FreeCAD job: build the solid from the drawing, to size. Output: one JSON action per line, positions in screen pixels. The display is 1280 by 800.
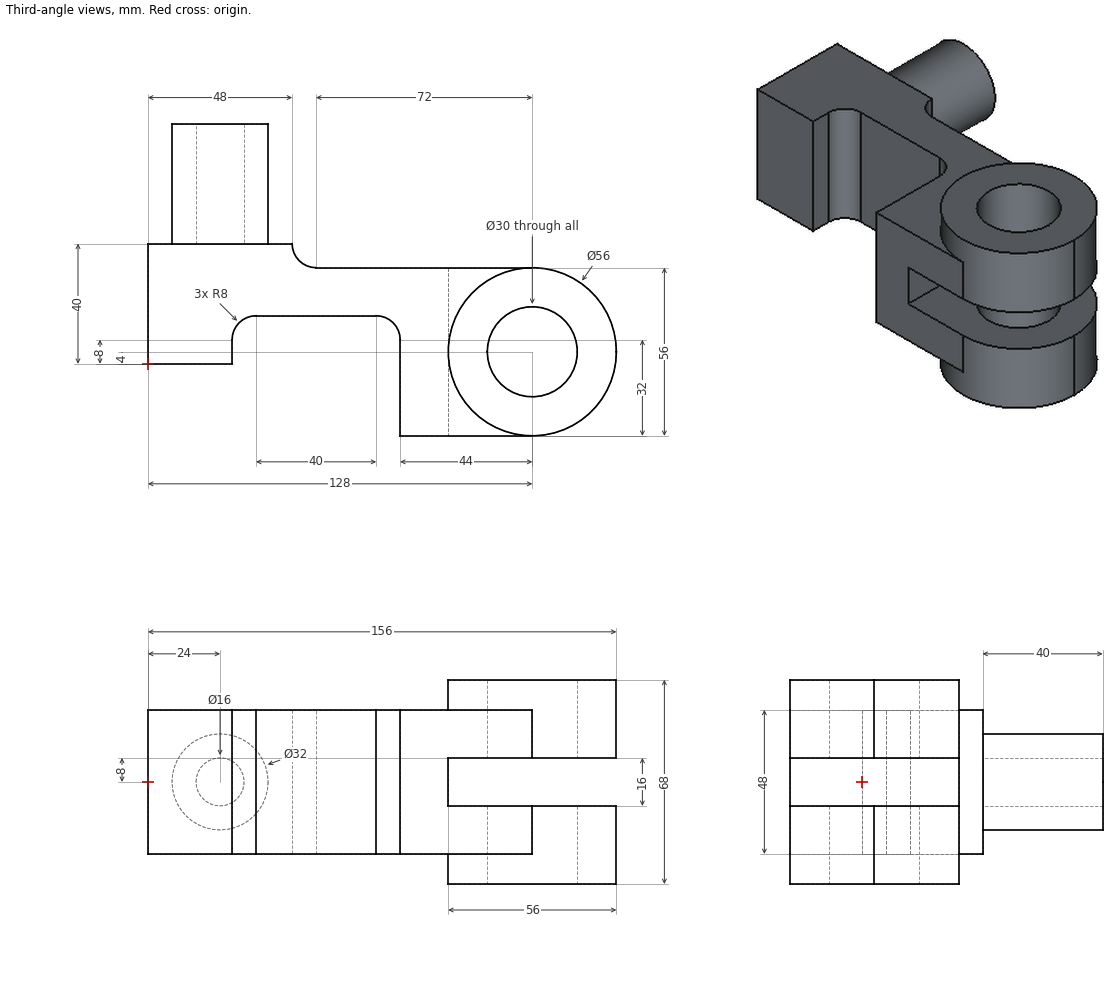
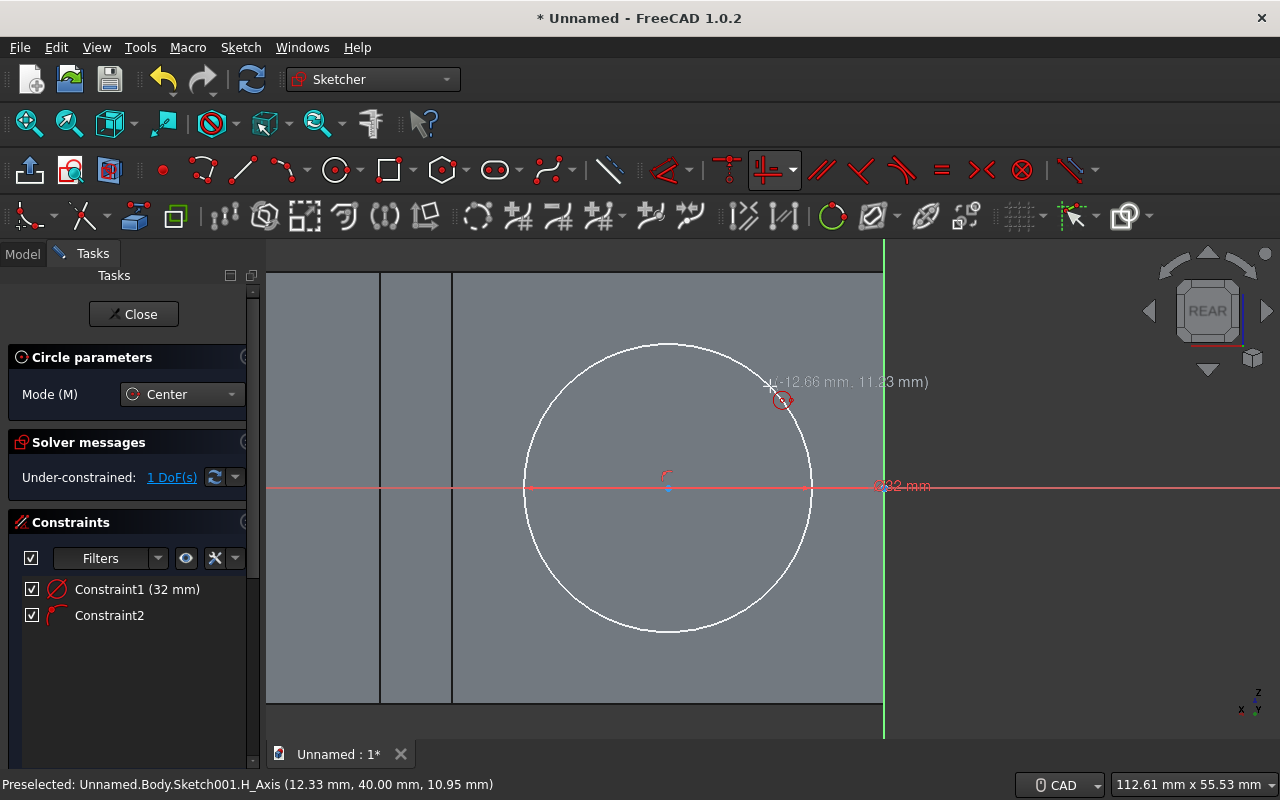
{"action": "left_click", "coordinate": [668, 488]}
{"action": "mouse_move", "coordinate": [719, 437]}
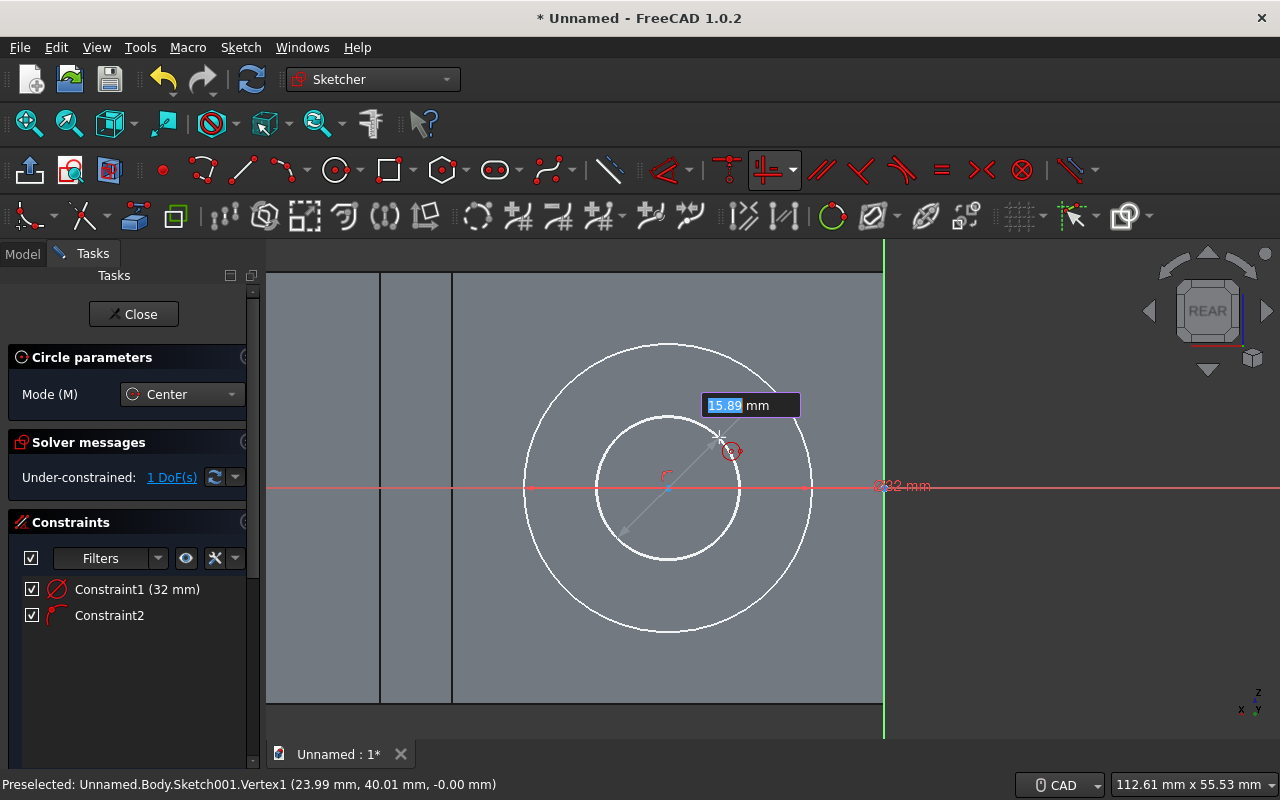
{"action": "type", "text": "16"}
{"action": "key", "text": "Return"}
{"action": "key", "text": "Escape"}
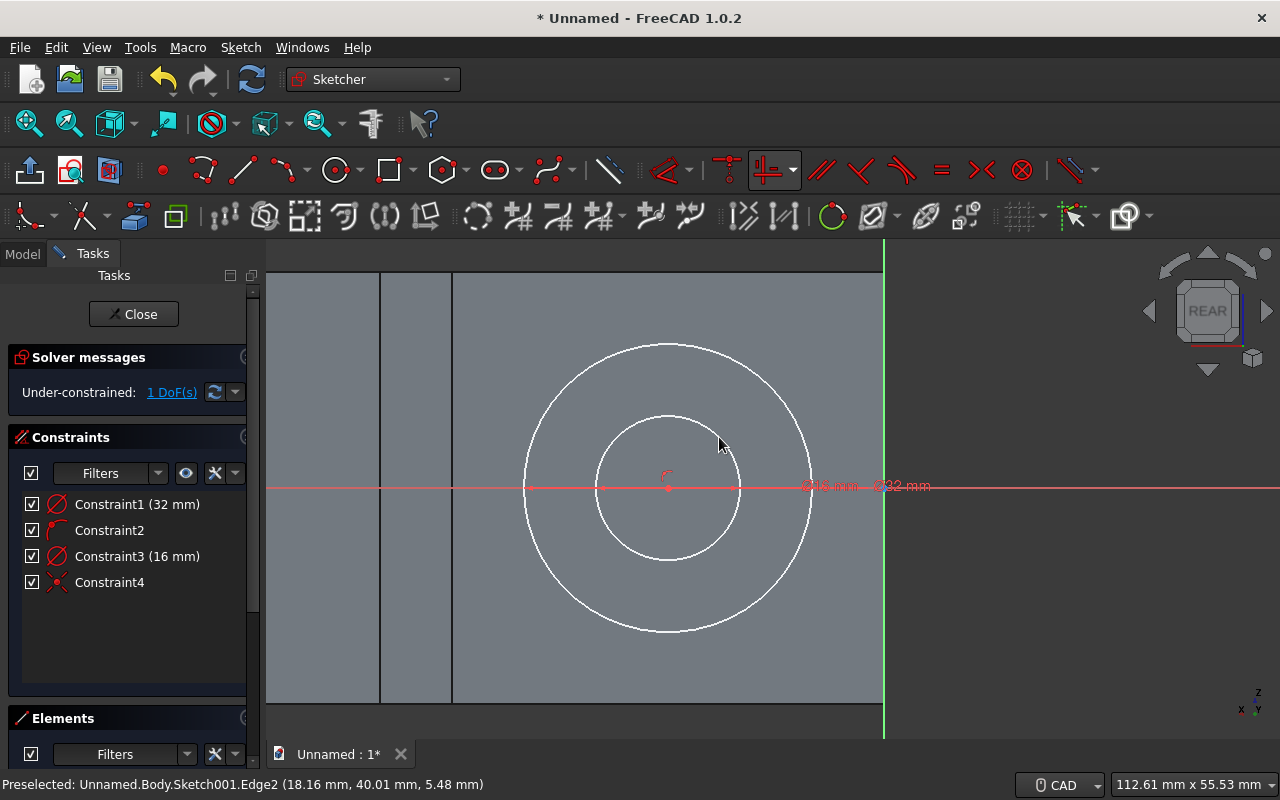
{"action": "left_click", "coordinate": [664, 170]}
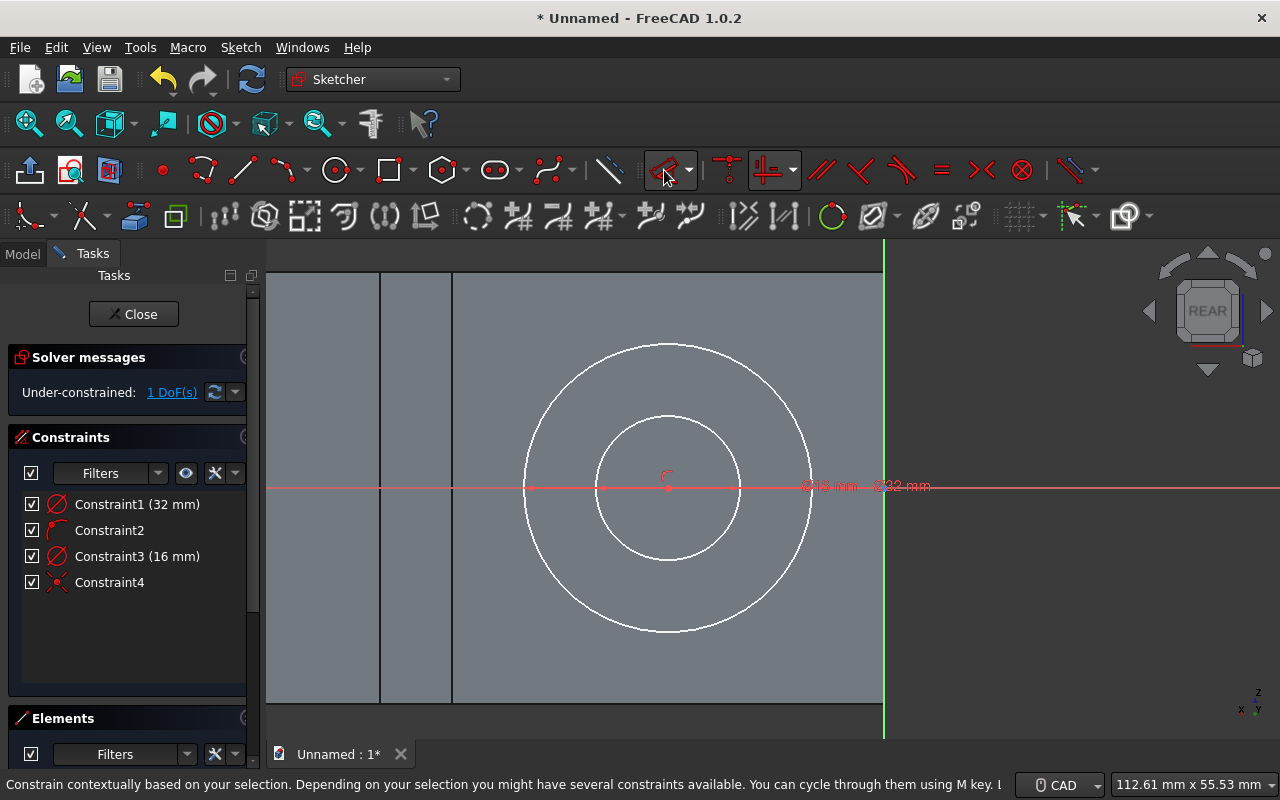
{"action": "left_click", "coordinate": [668, 488]}
{"action": "left_click", "coordinate": [776, 522]}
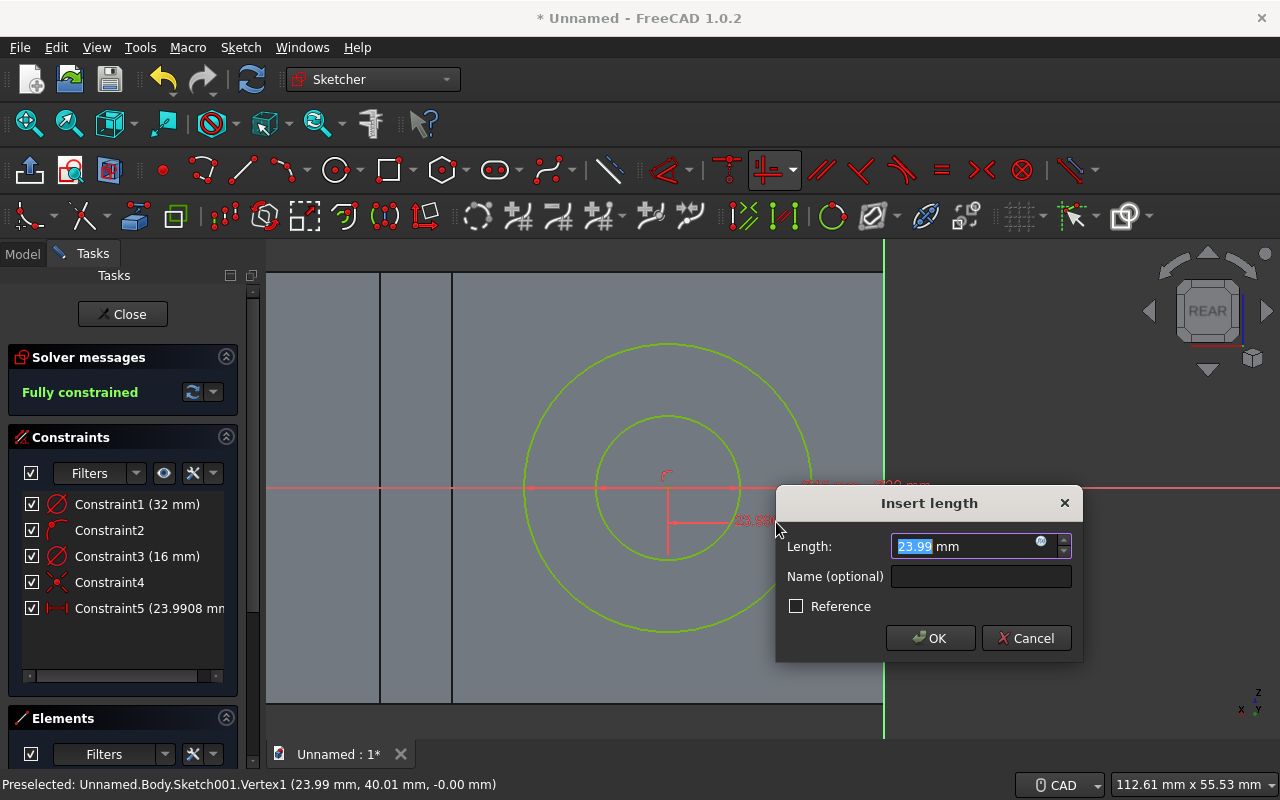
{"action": "type", "text": "24"}
{"action": "key", "text": "Return"}
{"action": "key", "text": "Escape"}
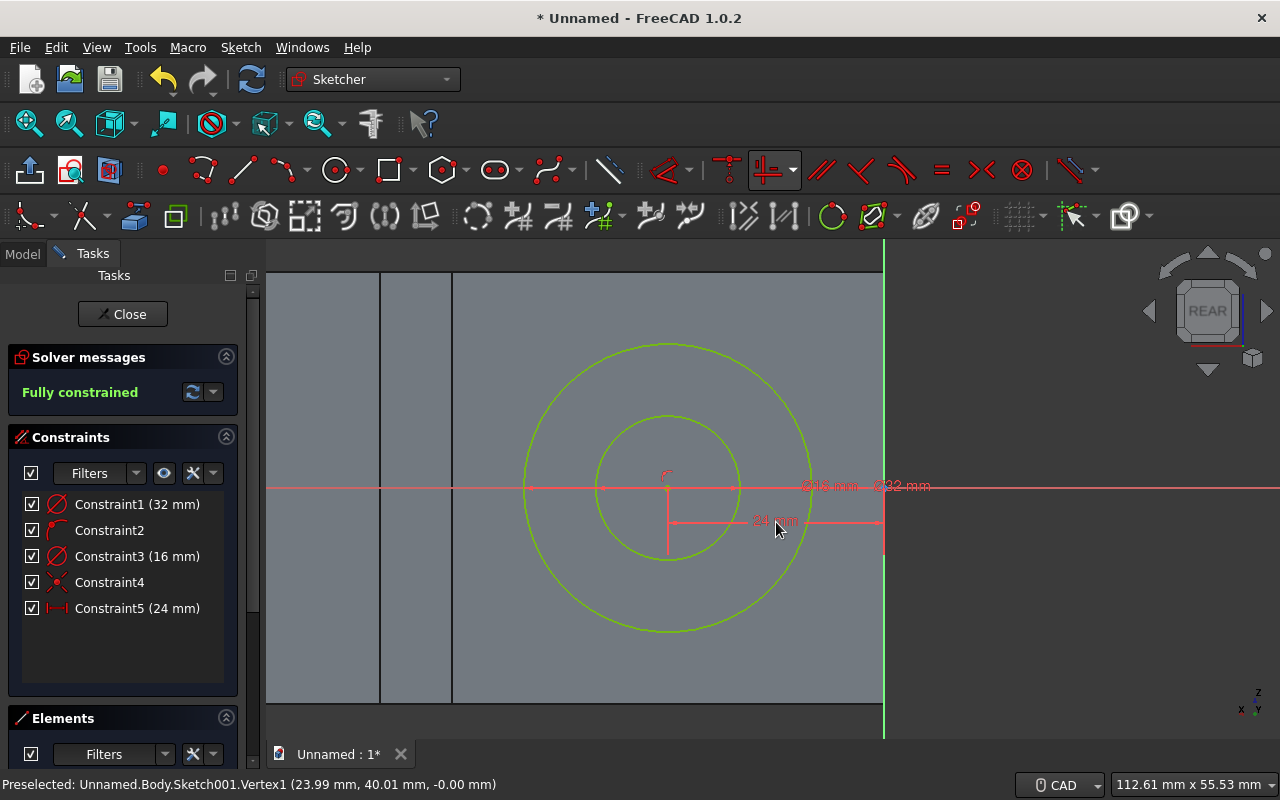
{"action": "left_click", "coordinate": [123, 314]}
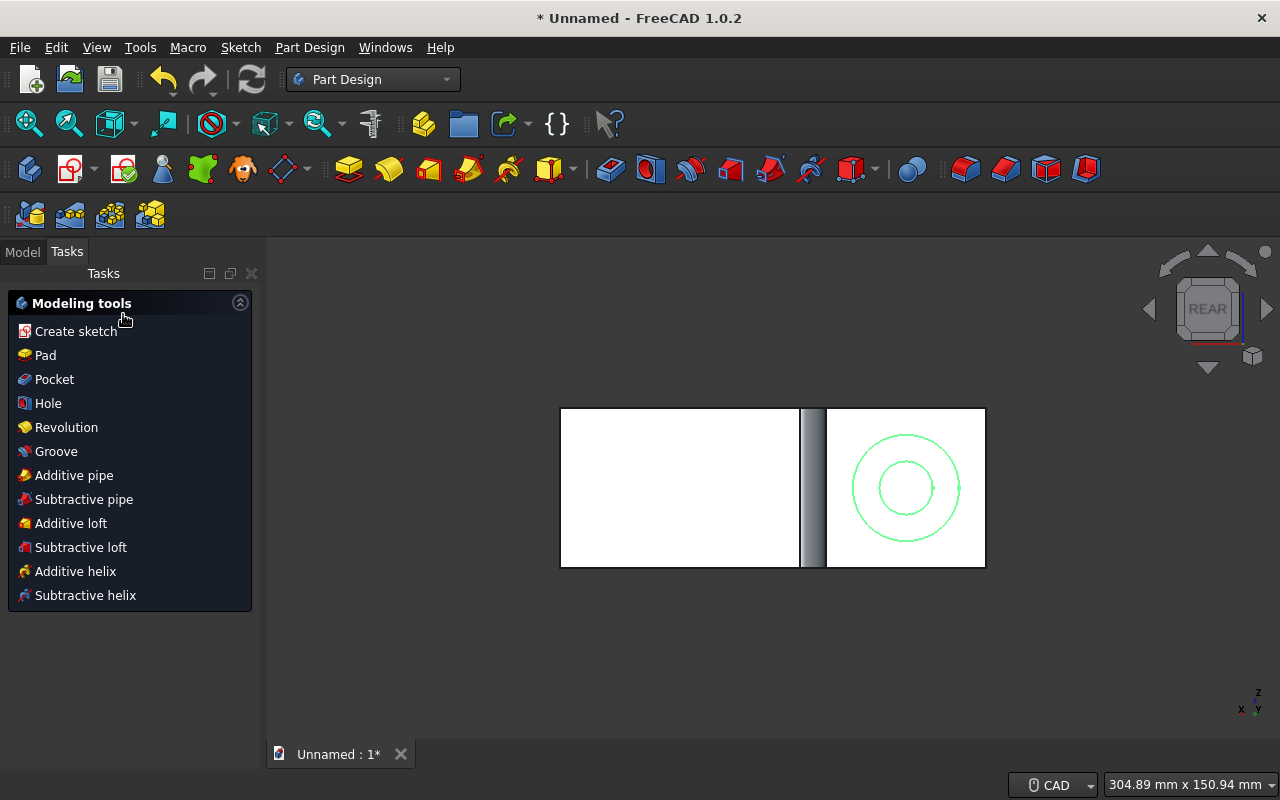
{"action": "left_click", "coordinate": [350, 170]}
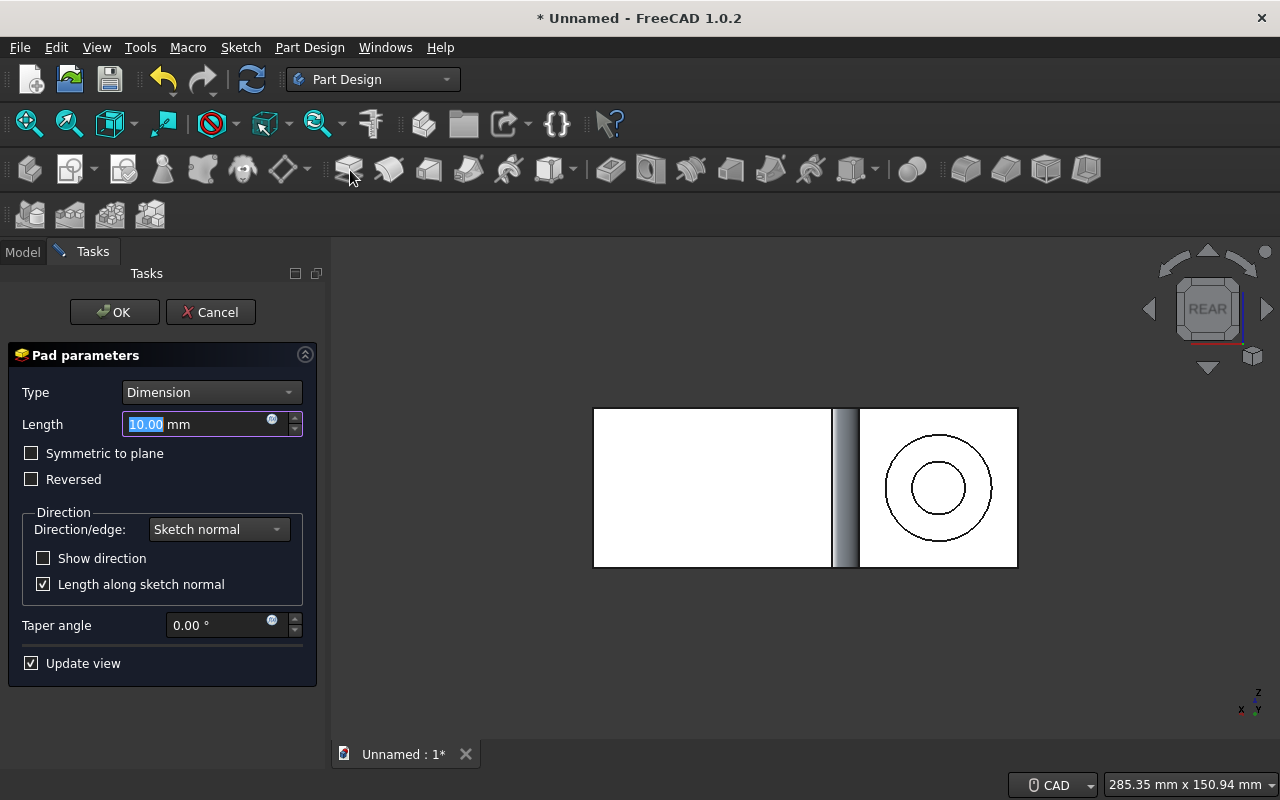
{"action": "type", "text": "40"}
{"action": "key", "text": "Tab"}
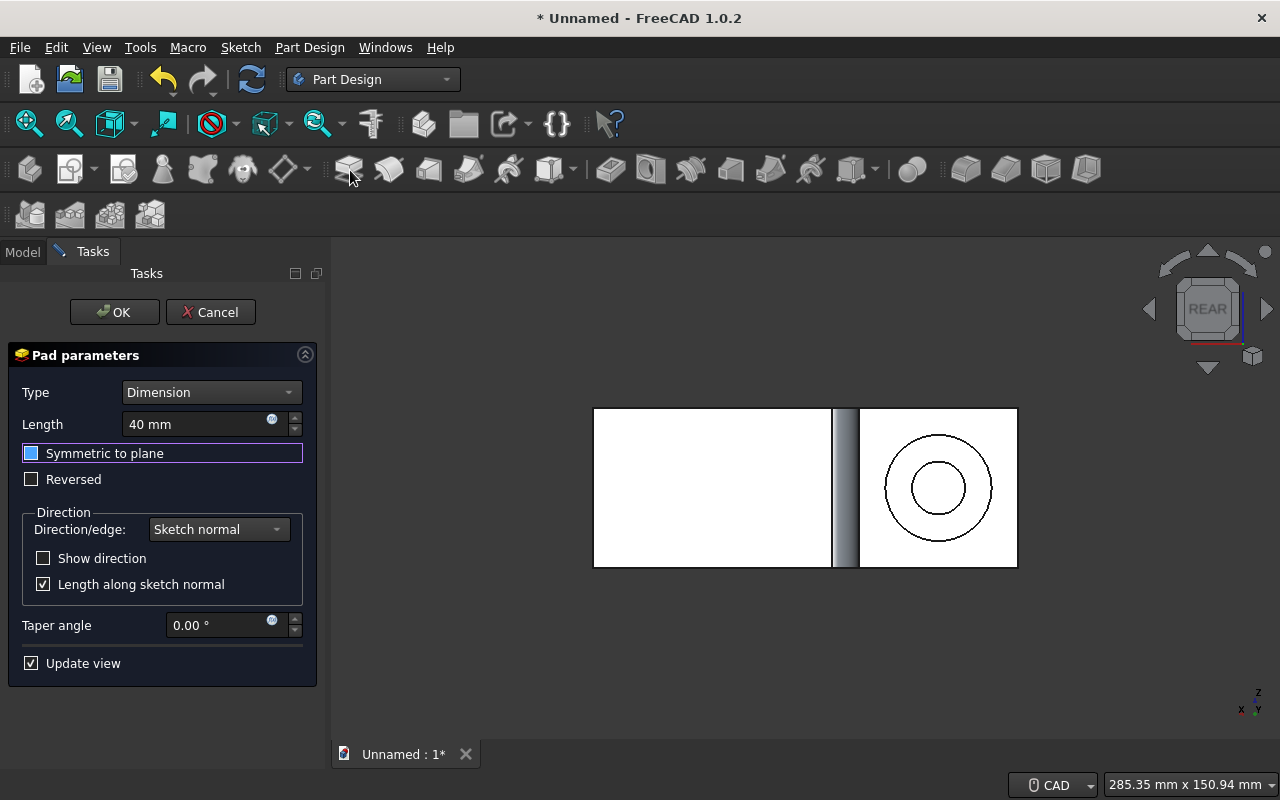
{"action": "left_click", "coordinate": [115, 312]}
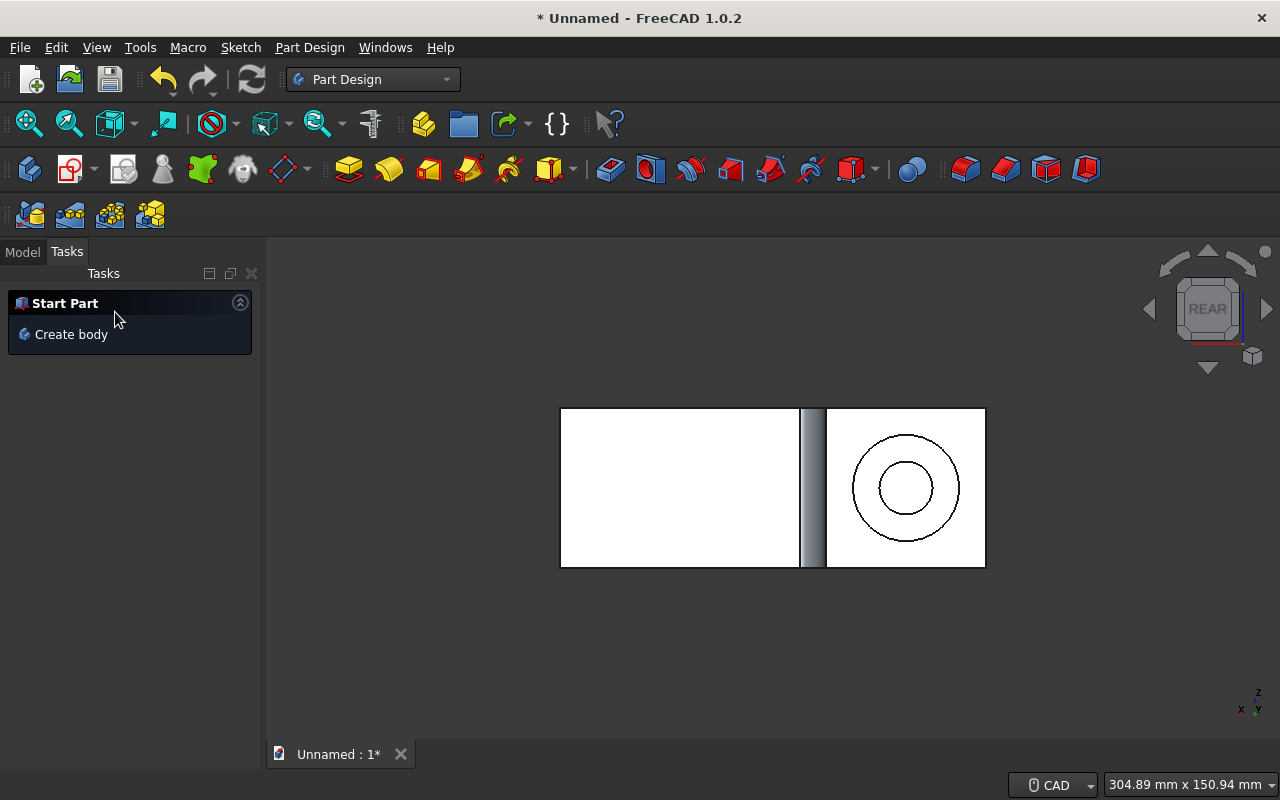
{"action": "key", "text": "v f"}